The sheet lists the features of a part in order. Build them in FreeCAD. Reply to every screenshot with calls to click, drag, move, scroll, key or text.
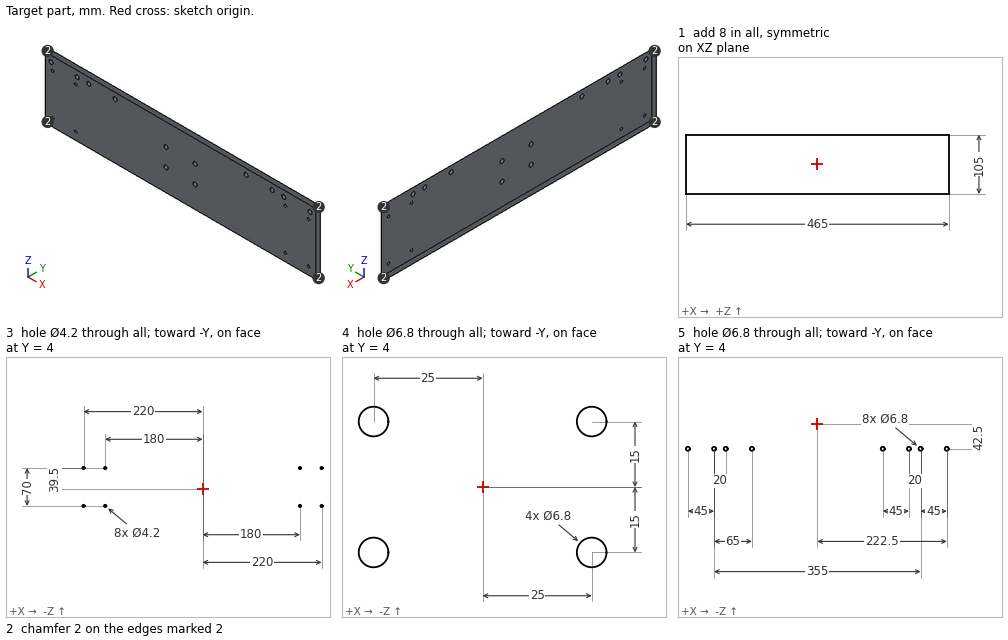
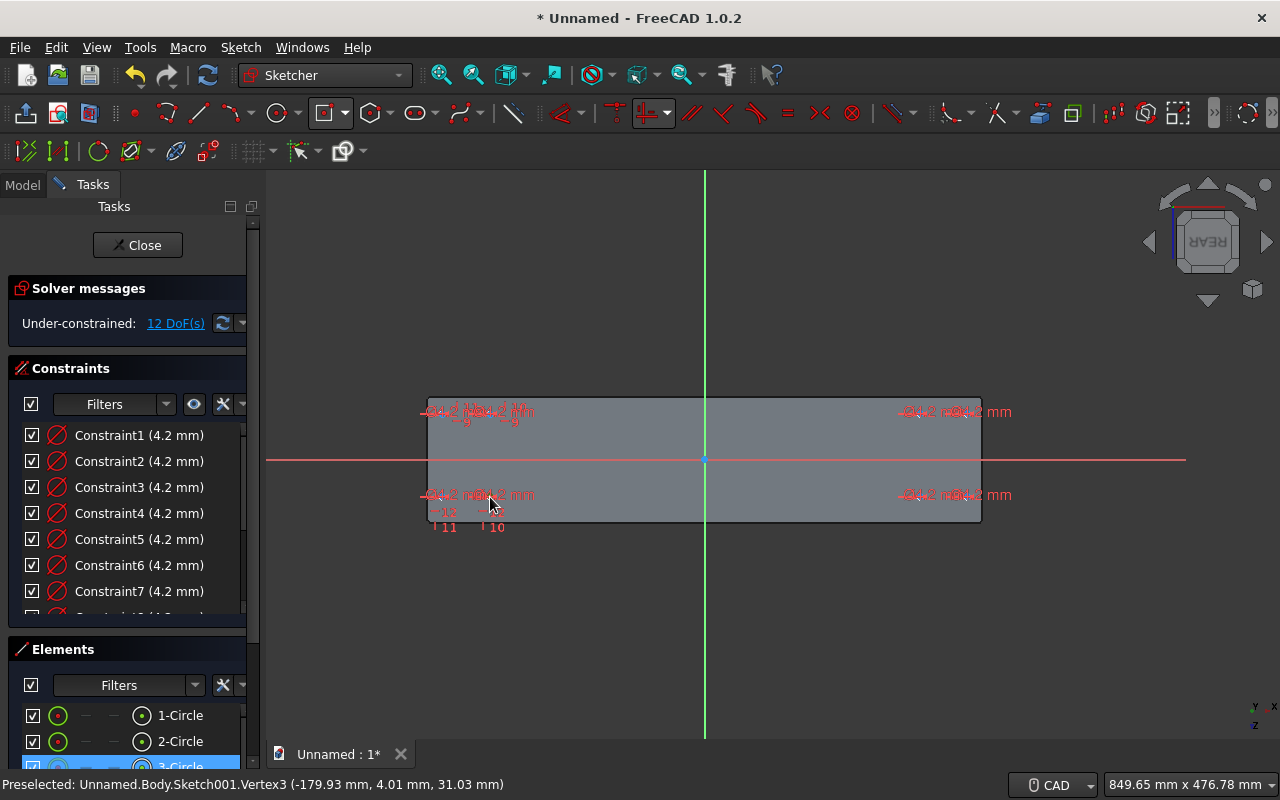
click(967, 497)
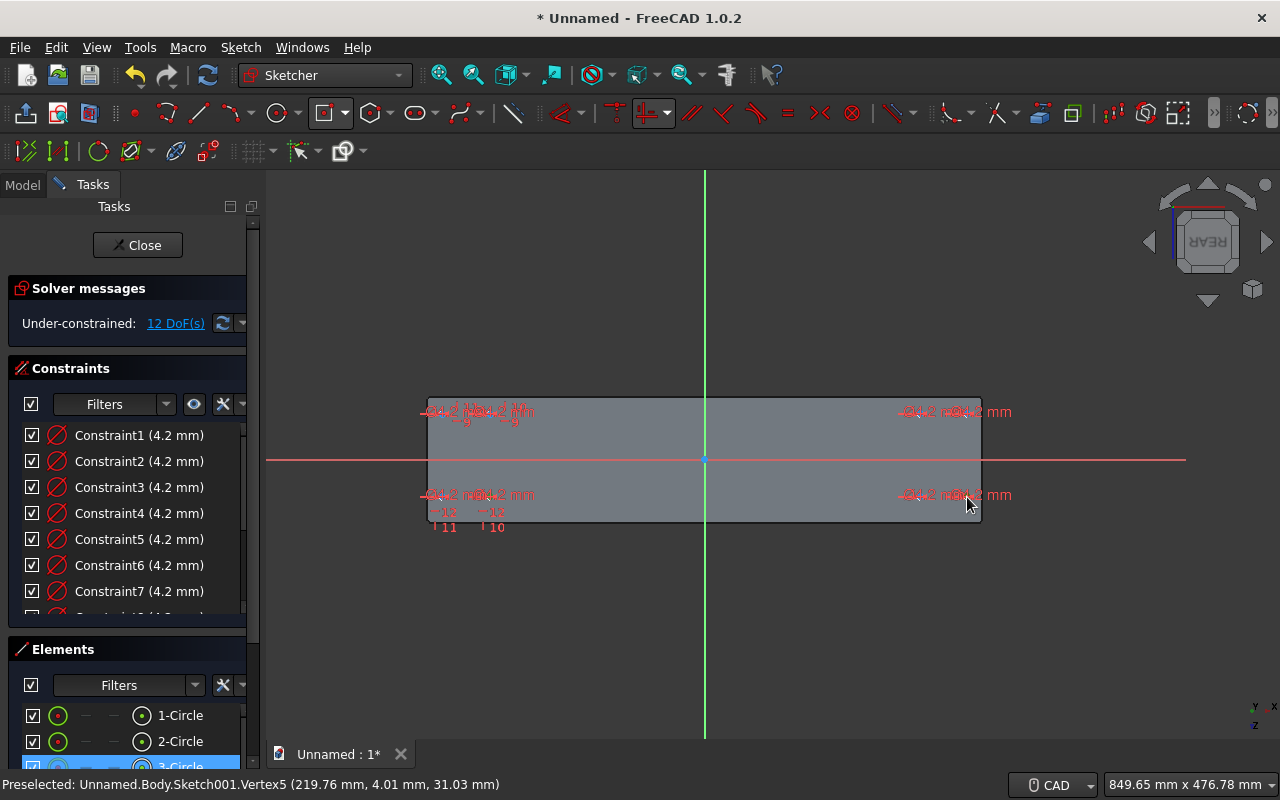
click(670, 114)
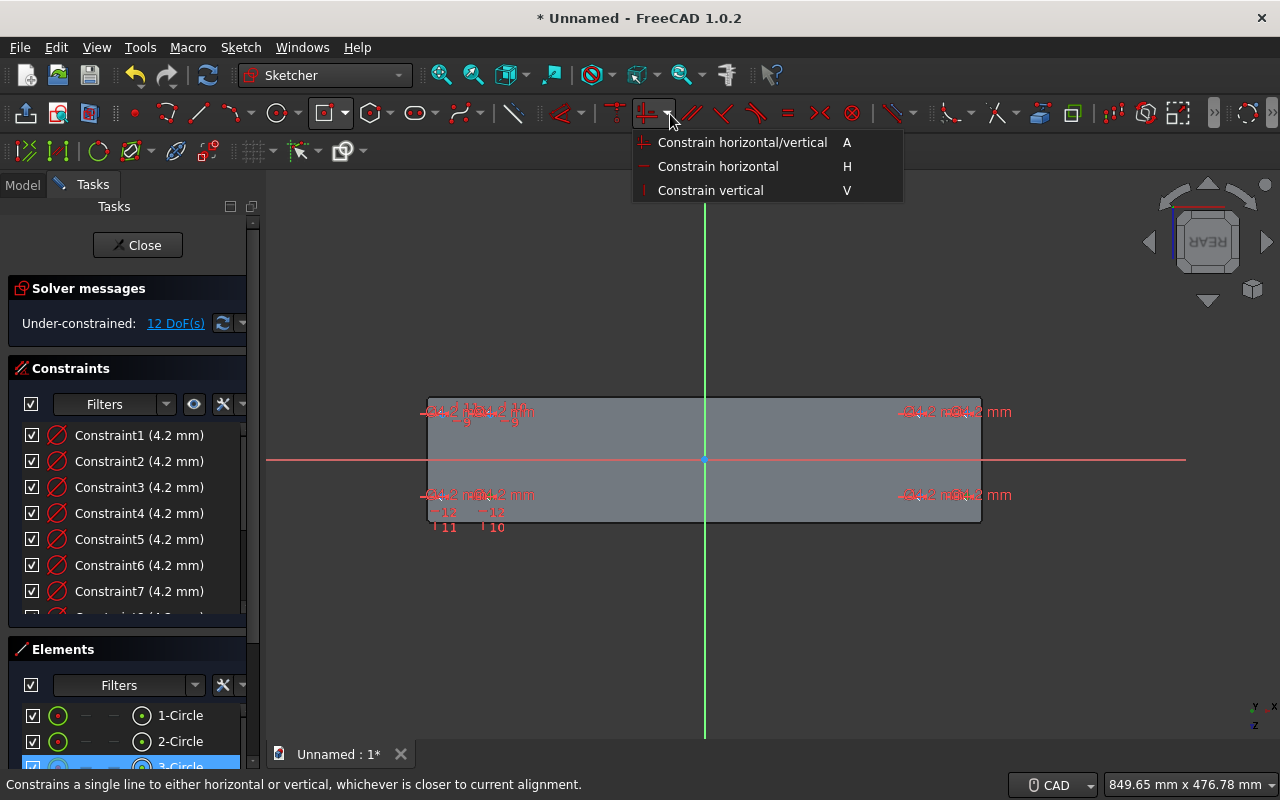
click(768, 166)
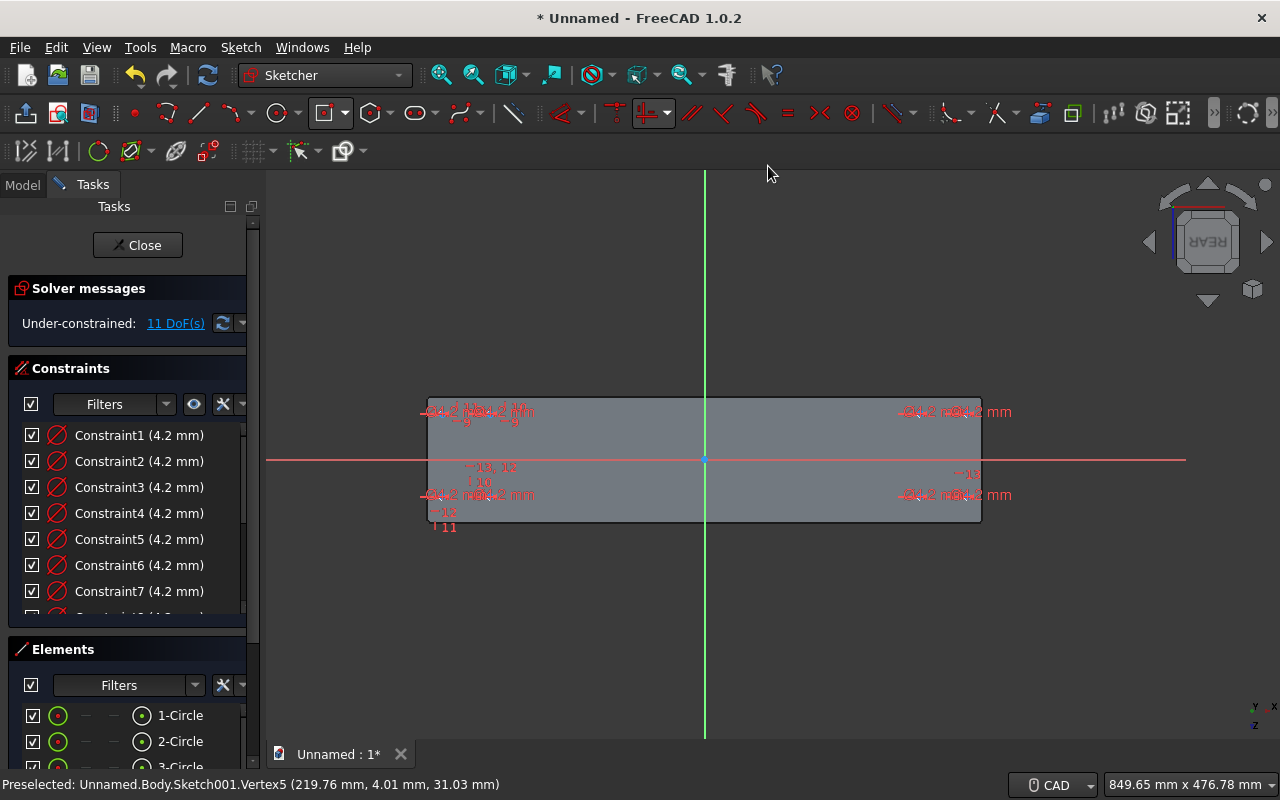
click(967, 497)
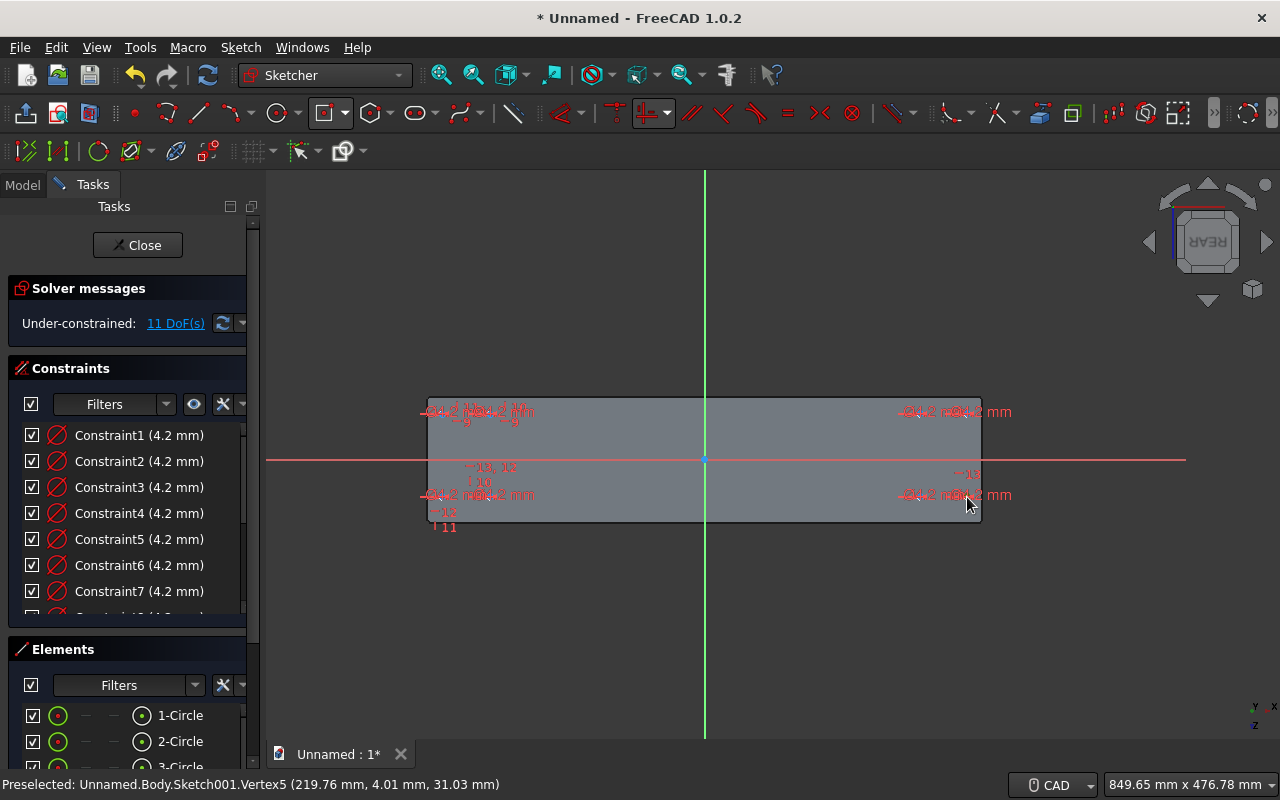
click(920, 497)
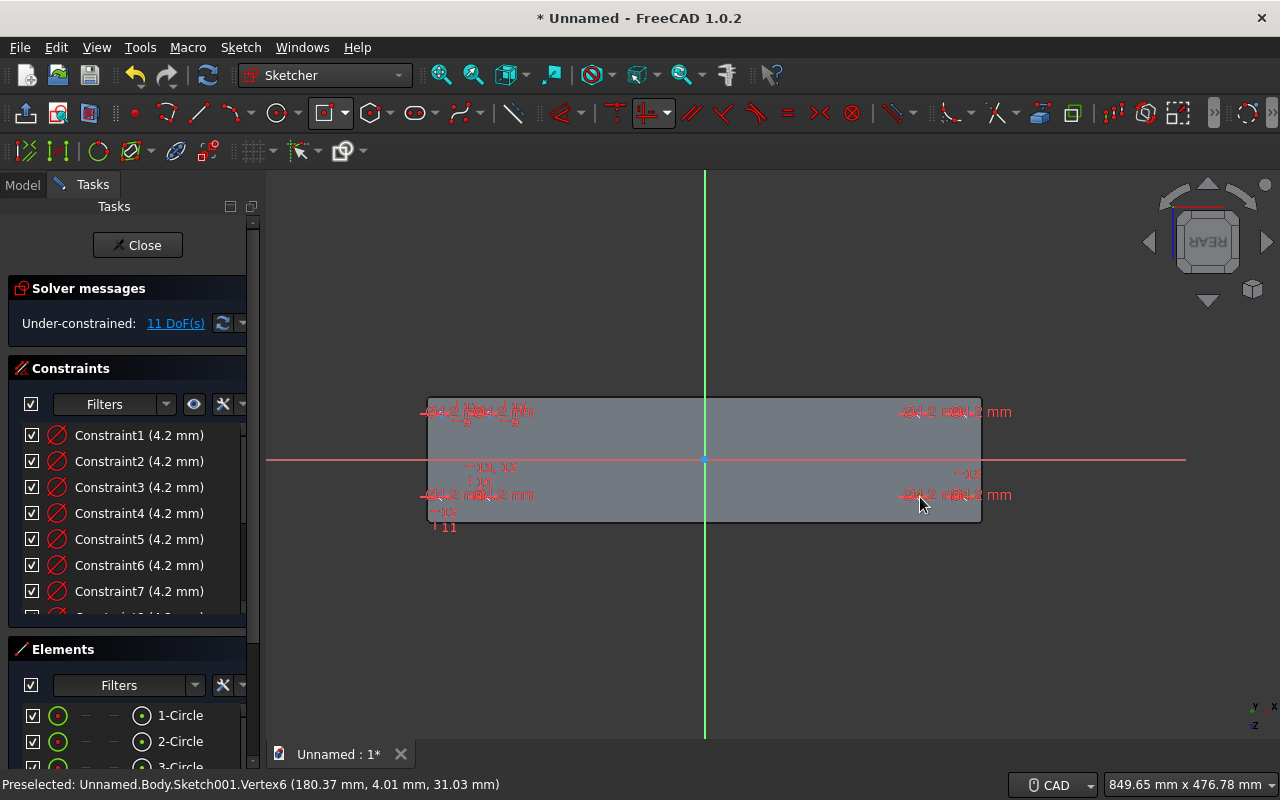
click(670, 114)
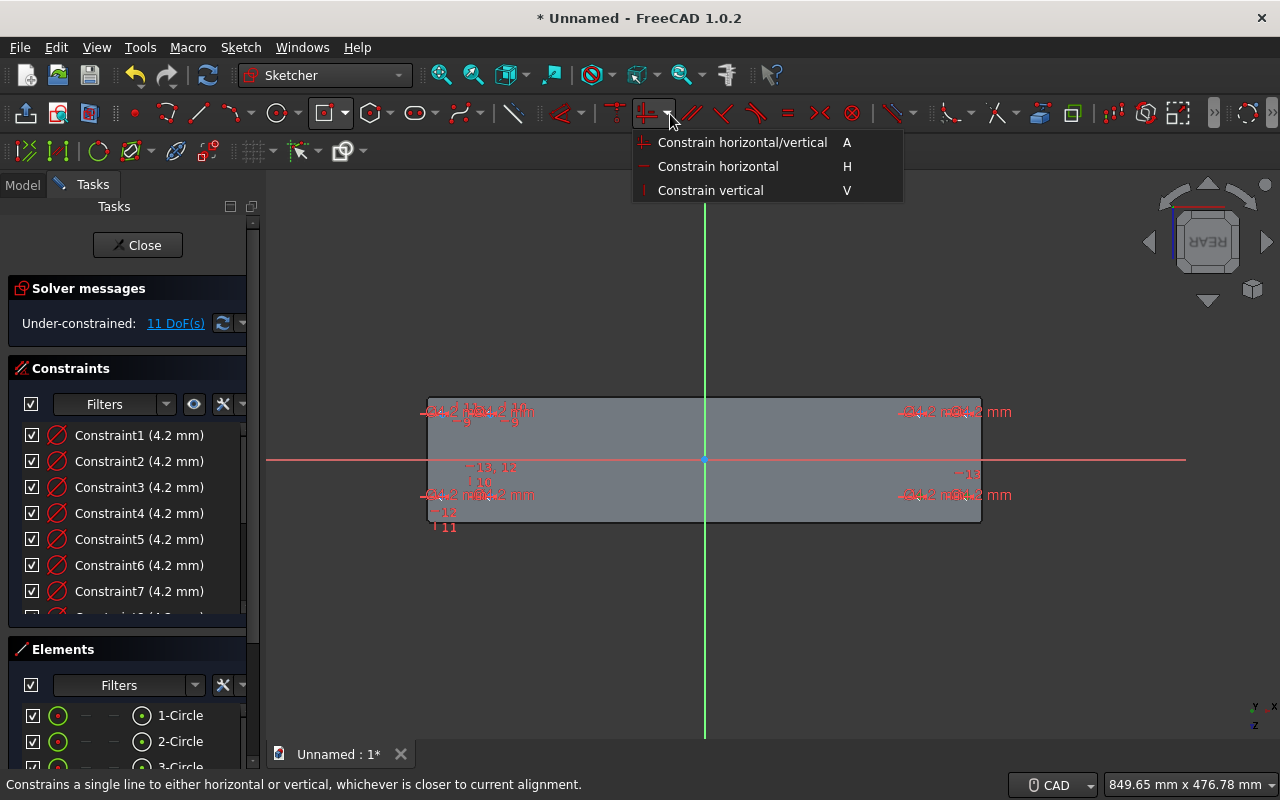
click(768, 166)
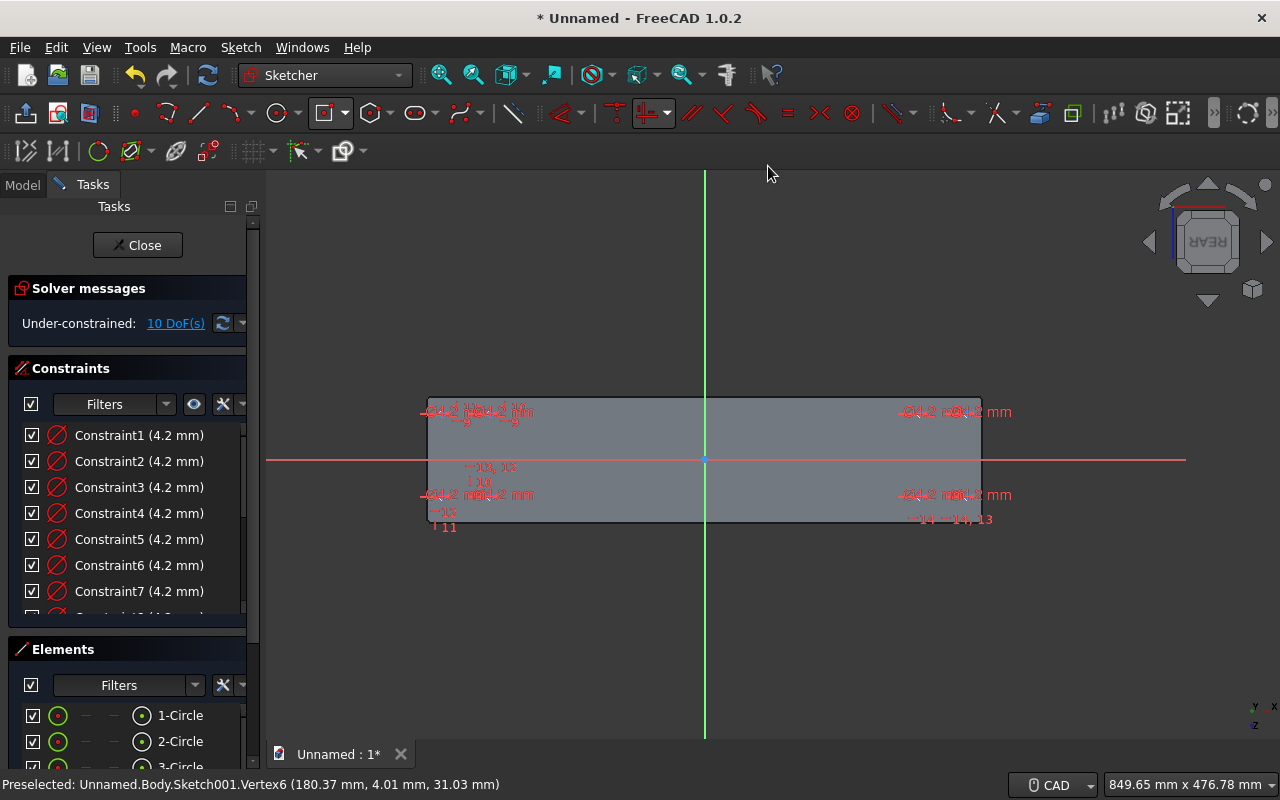
click(920, 497)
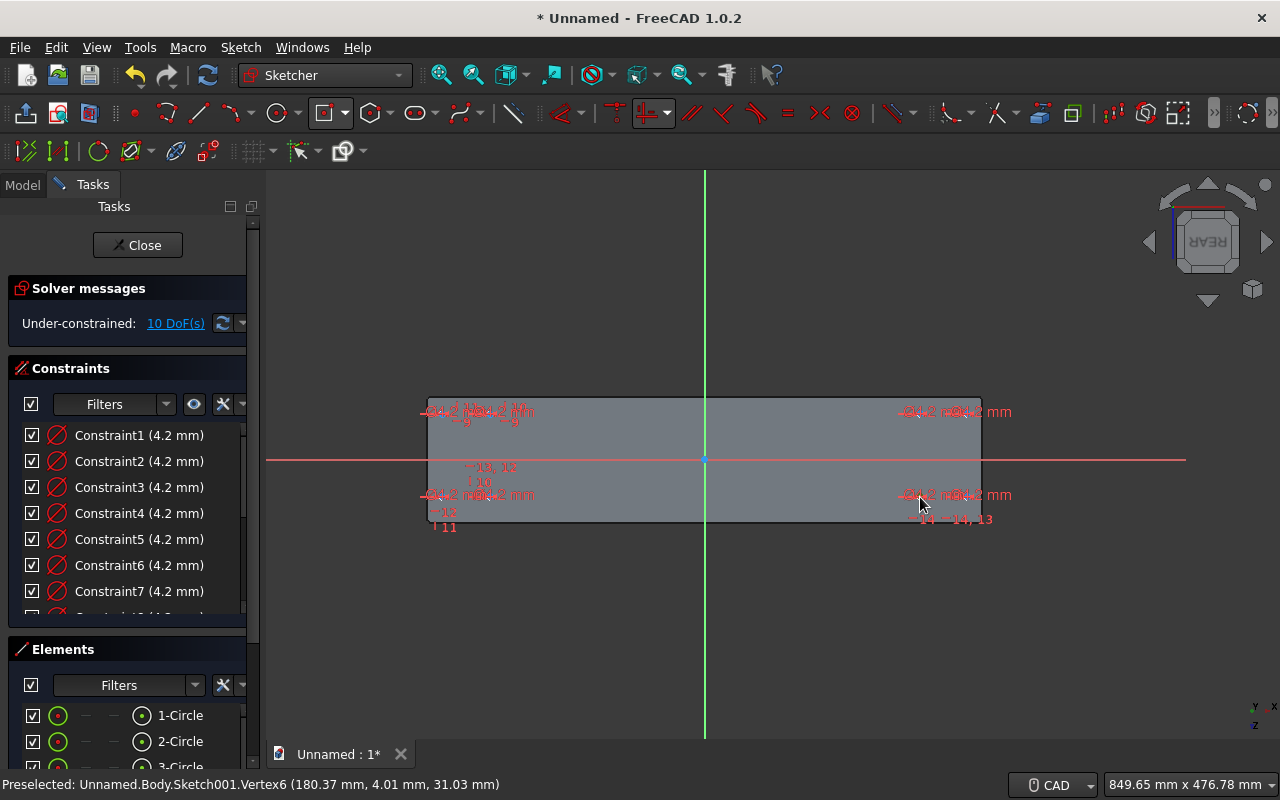
click(920, 414)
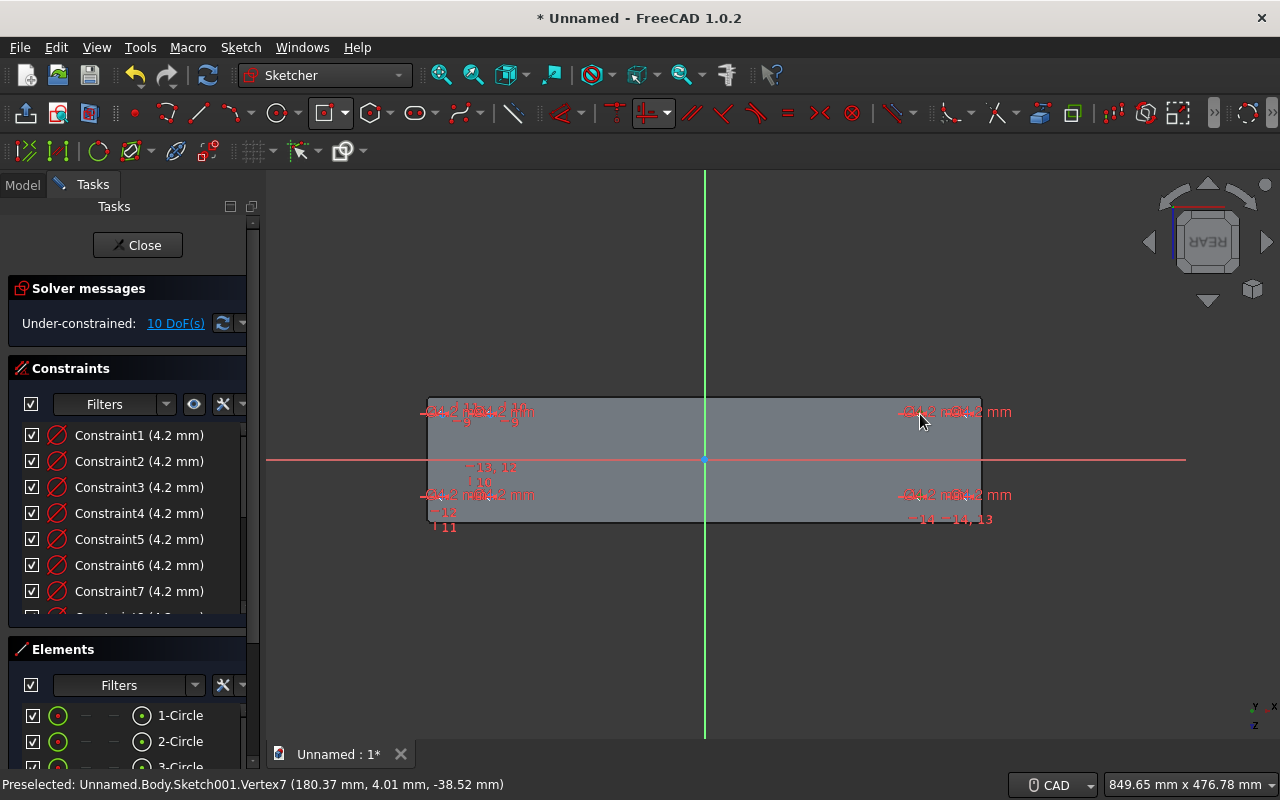
click(670, 114)